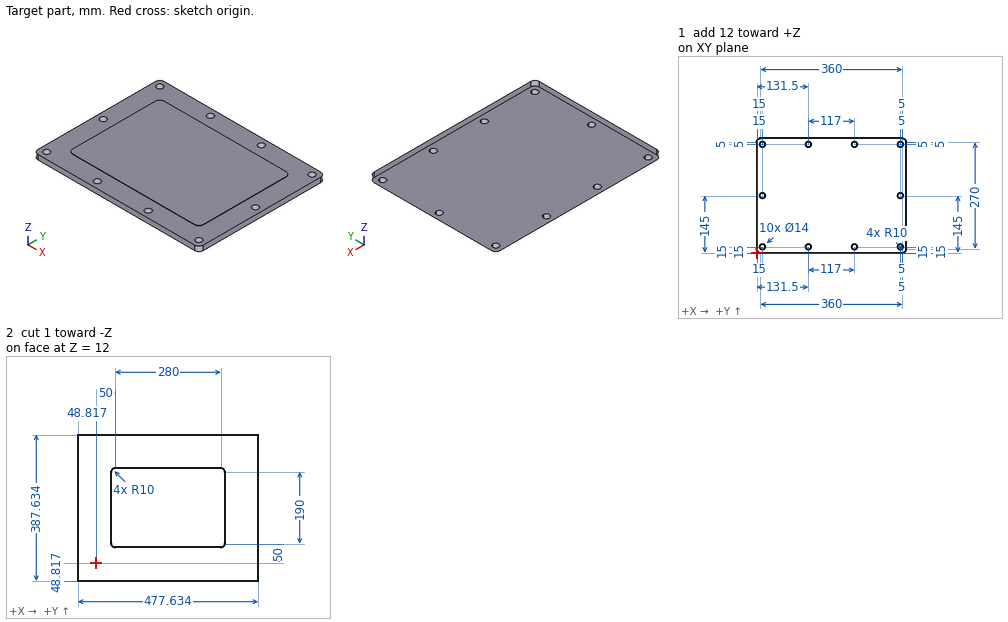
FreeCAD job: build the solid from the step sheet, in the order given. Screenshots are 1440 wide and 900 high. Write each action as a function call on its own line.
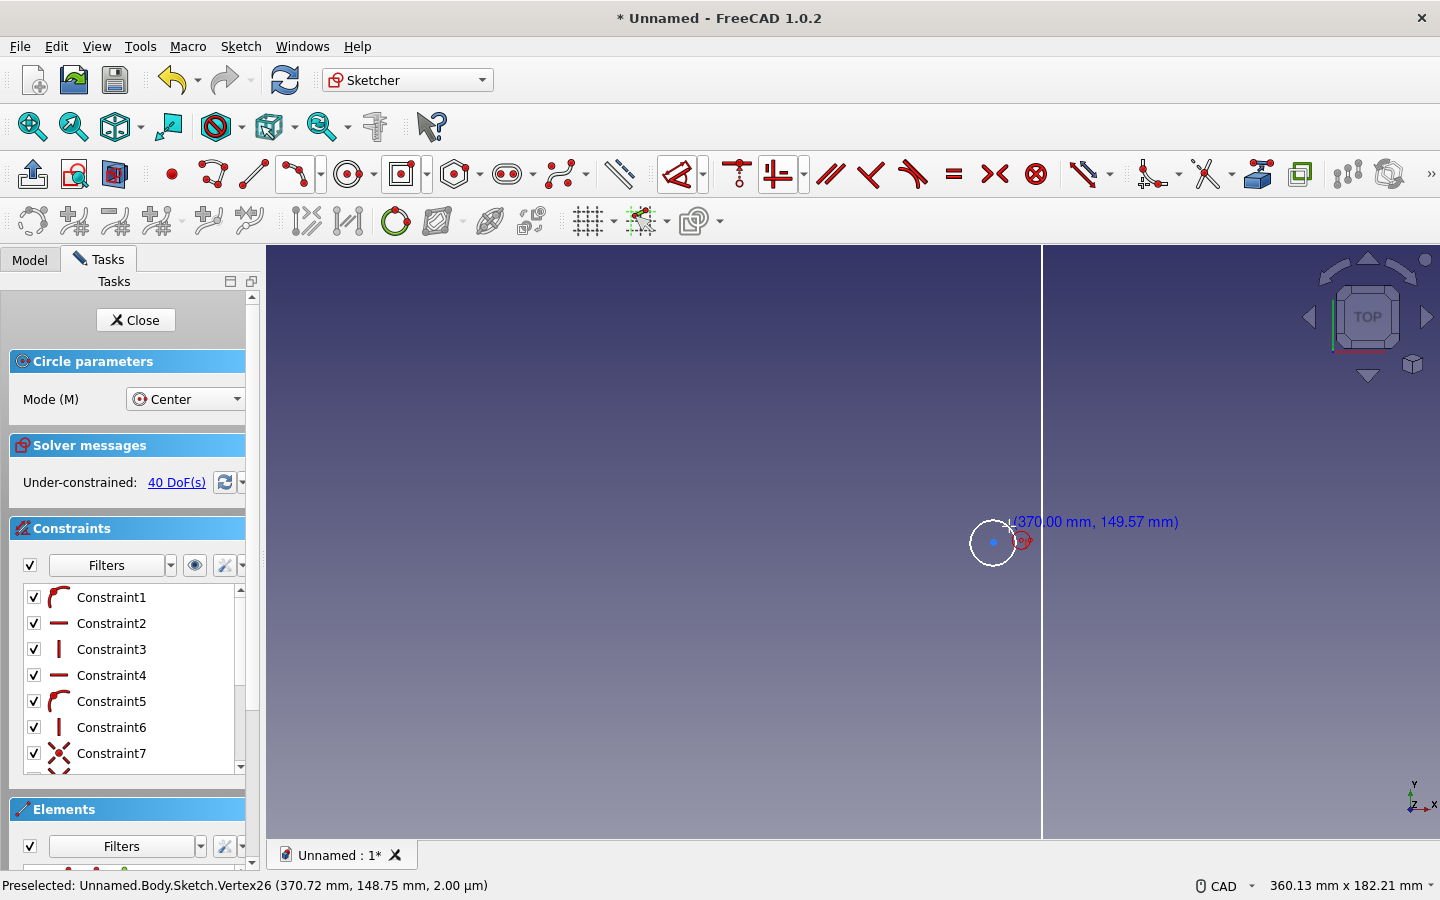
scroll(995, 542, down, 5)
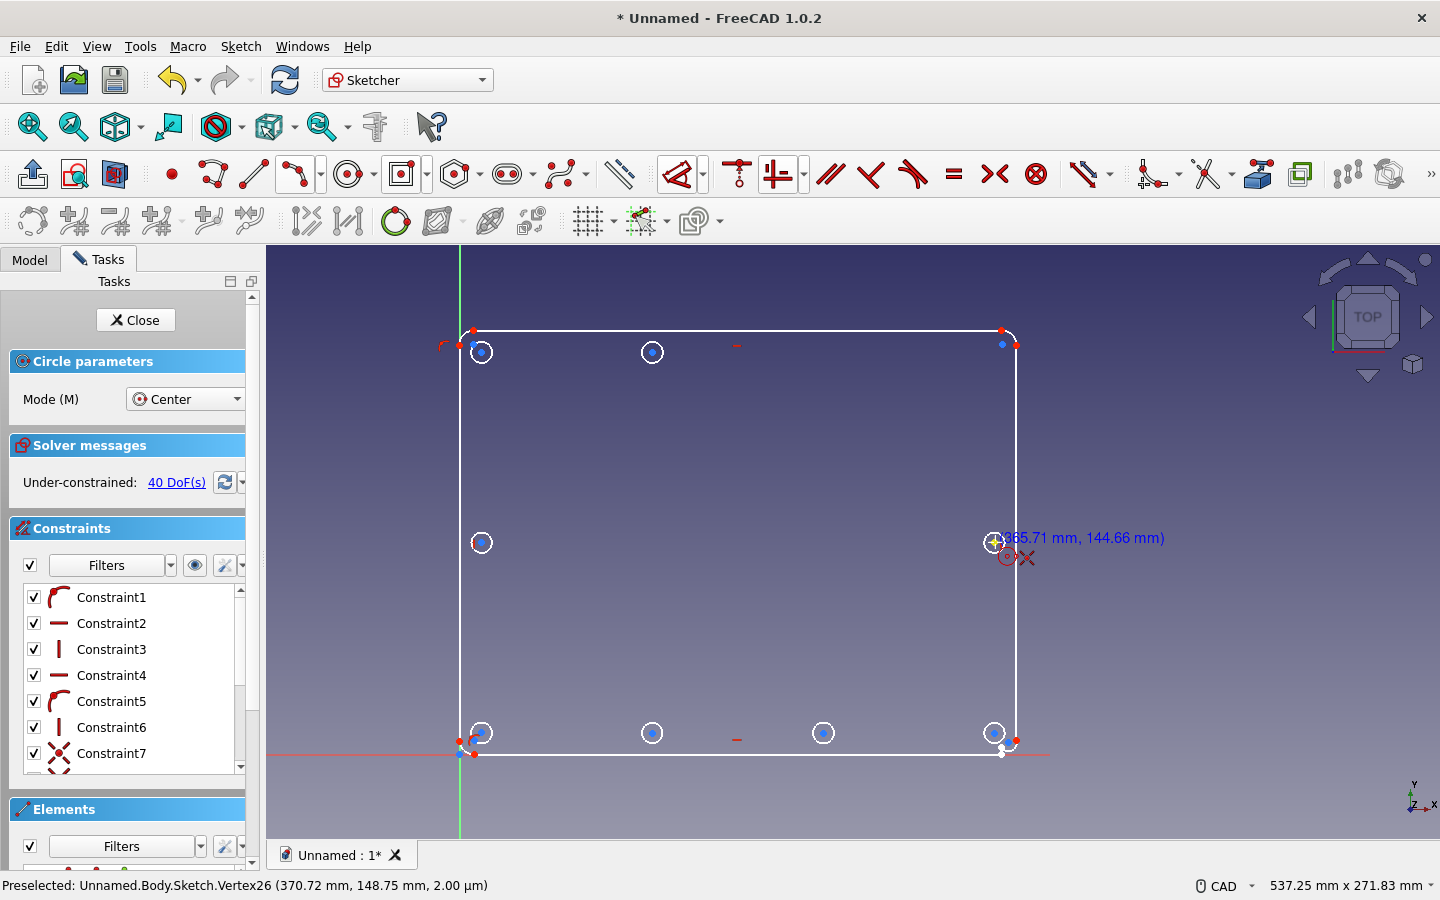
scroll(855, 386, up, 5)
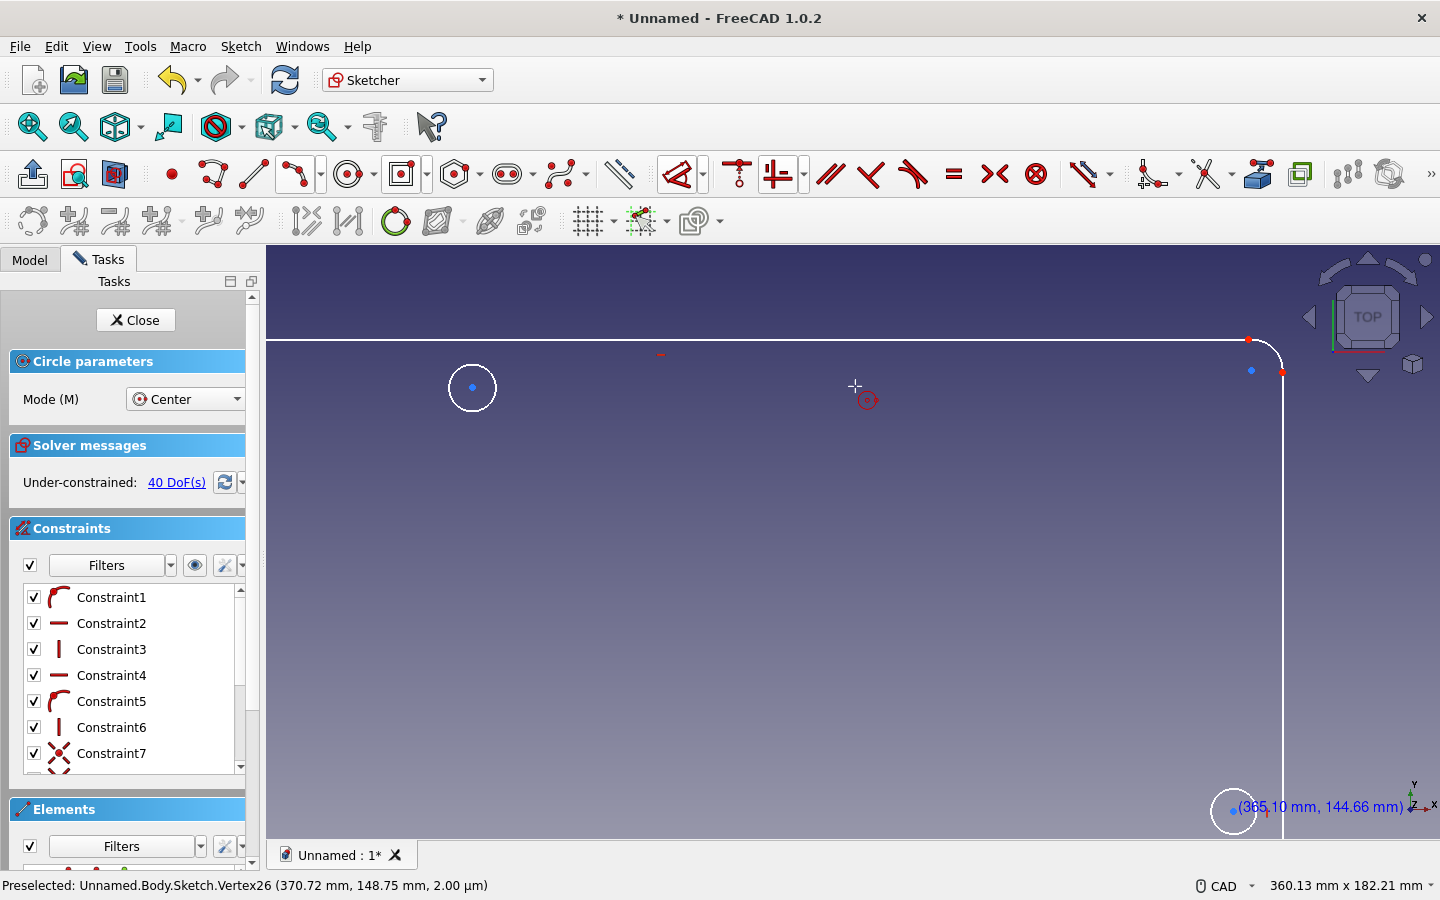
click(854, 387)
click(870, 370)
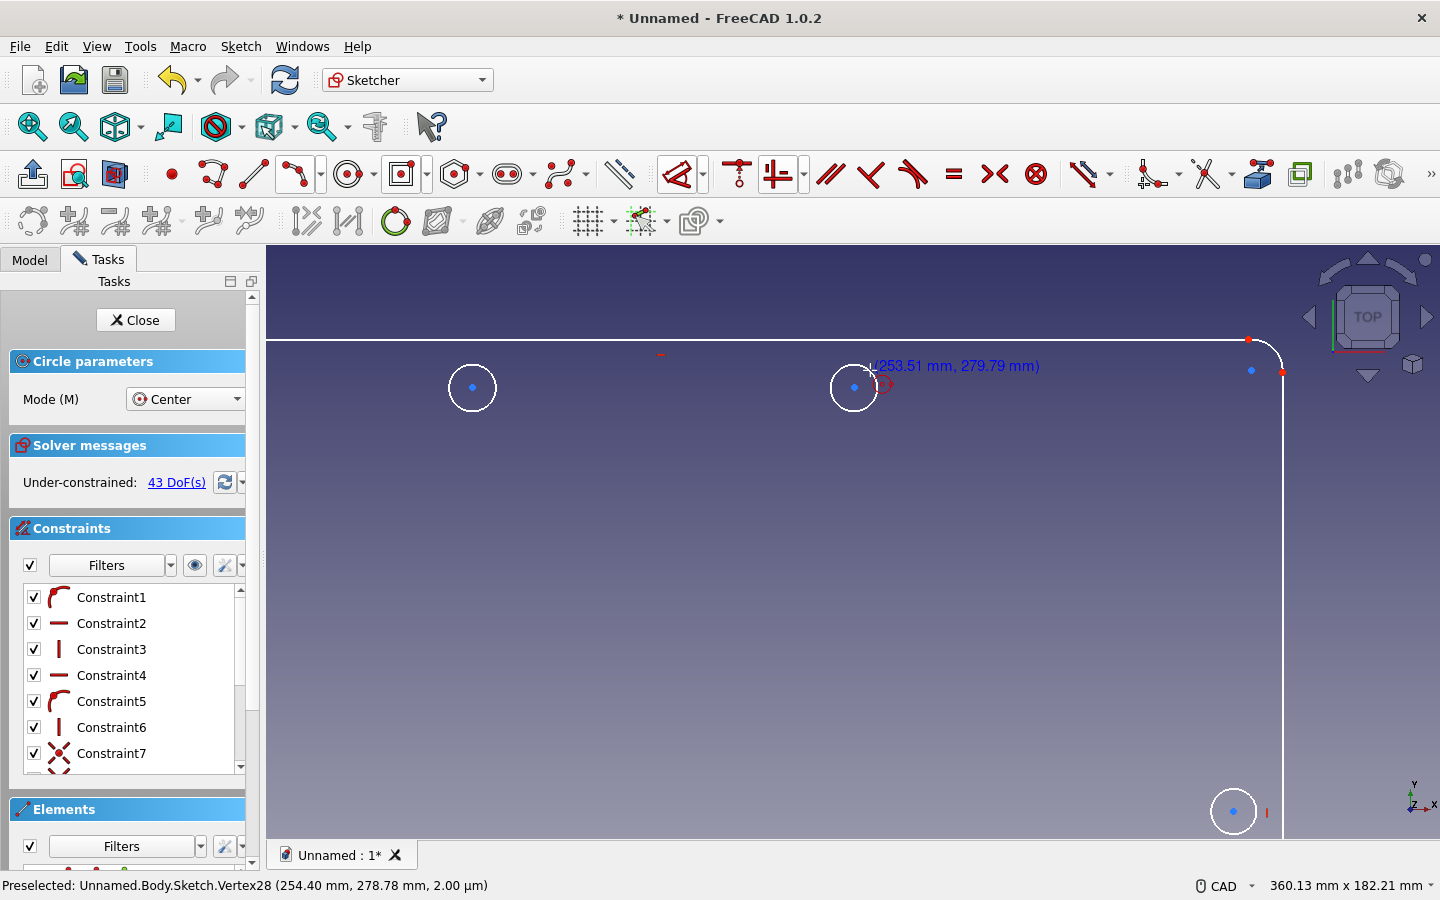
click(1233, 387)
click(1217, 370)
key(Escape)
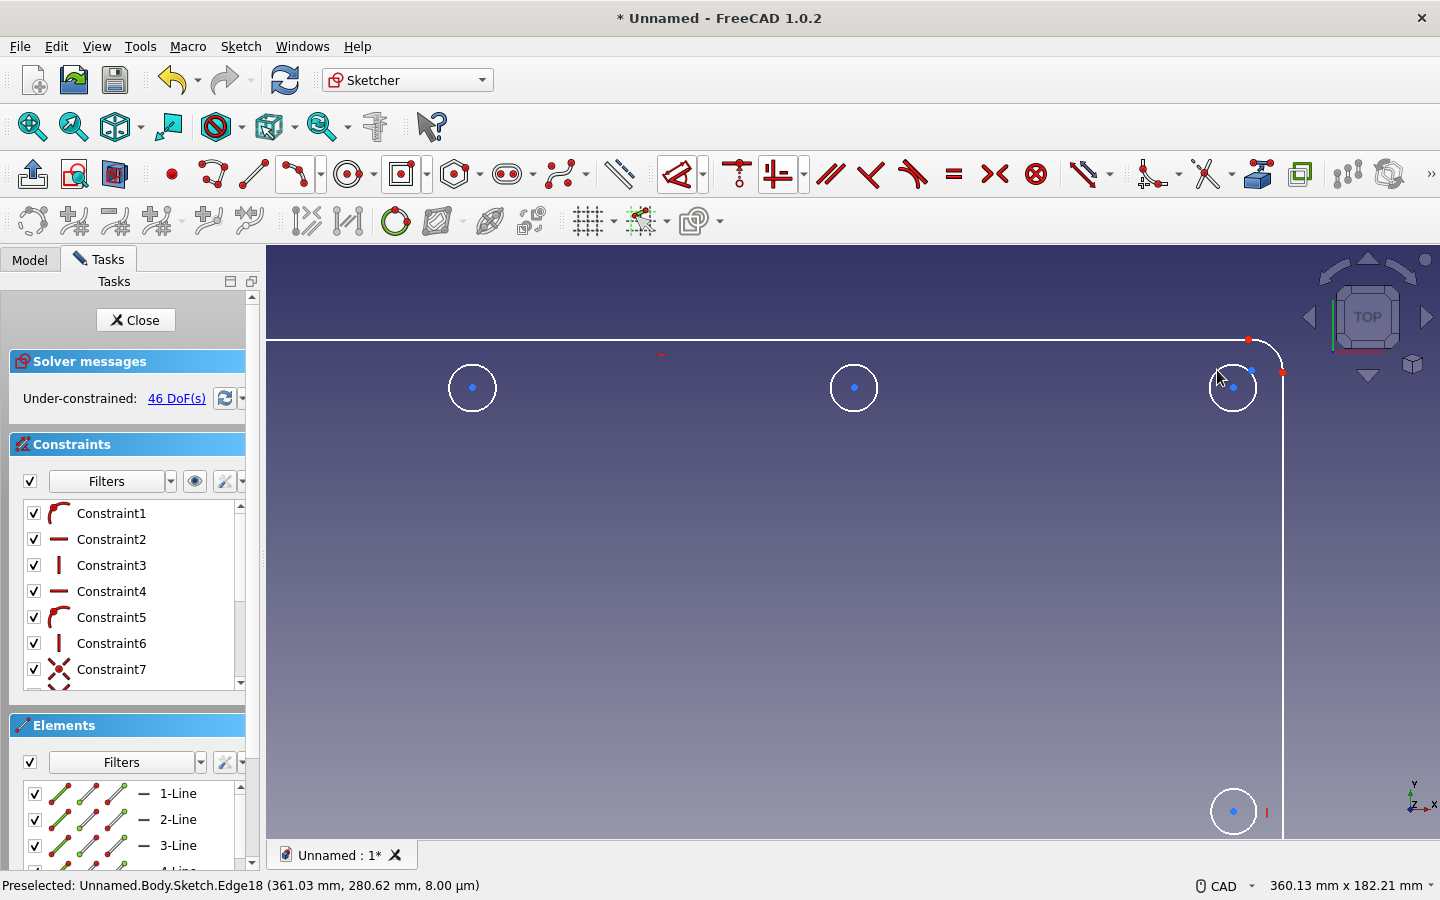
scroll(855, 386, down, 5)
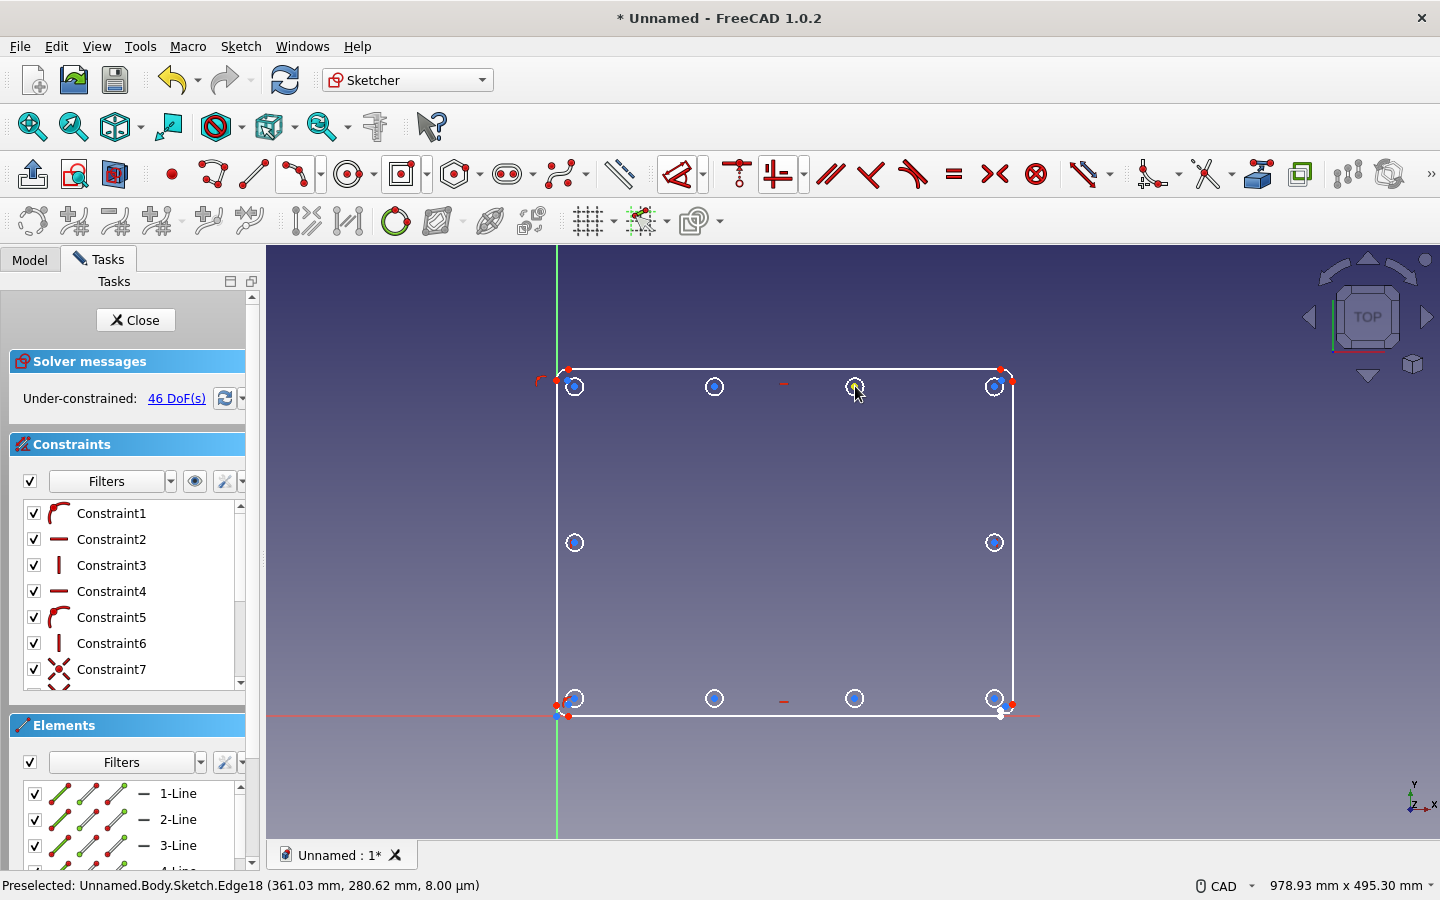
click(698, 716)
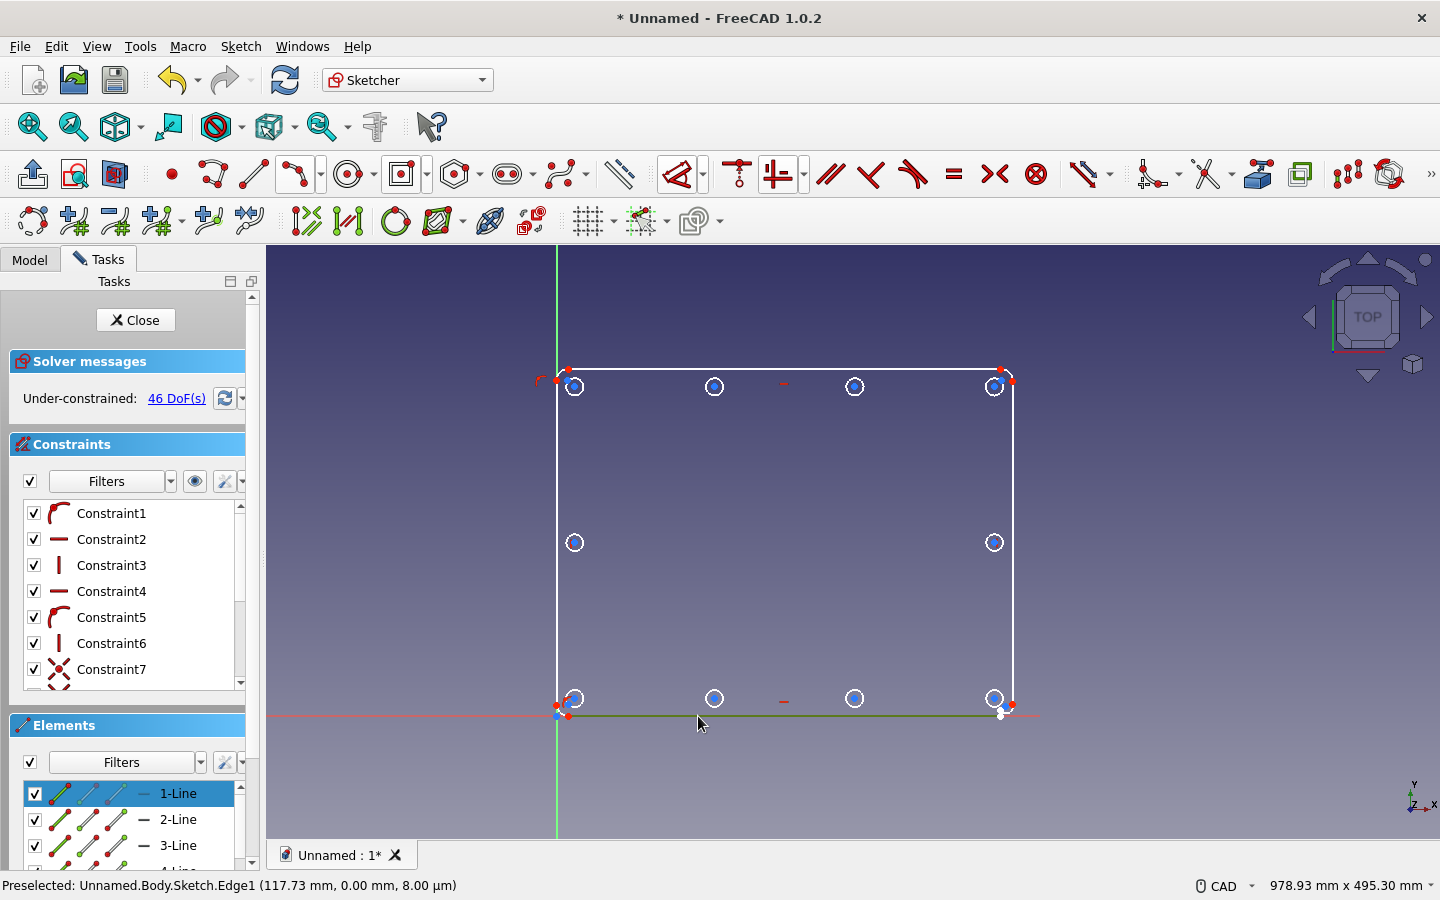
scroll(1009, 713, up, 4)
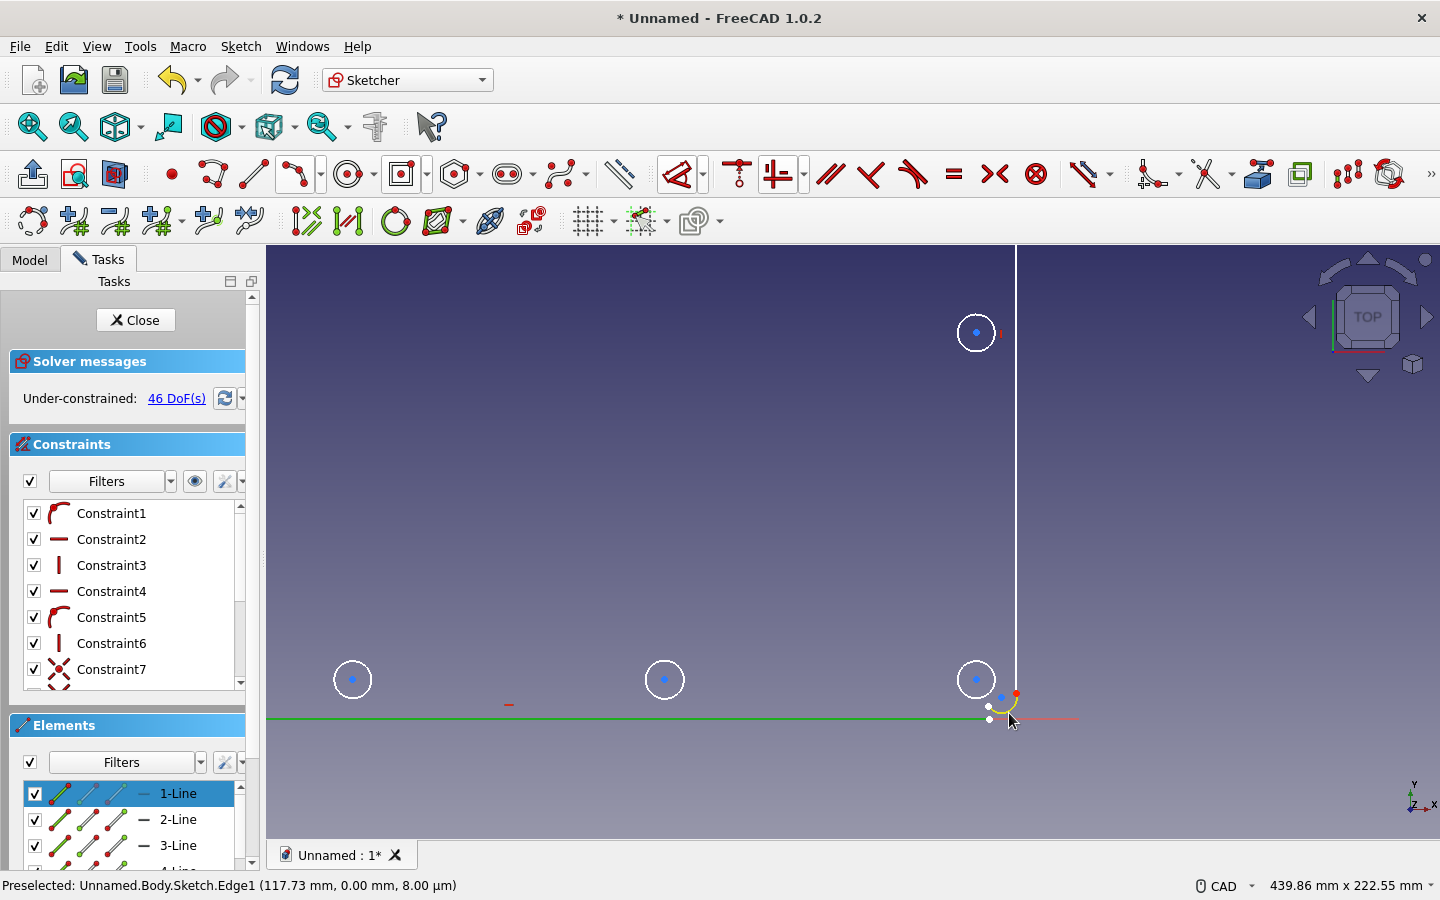
click(1008, 712)